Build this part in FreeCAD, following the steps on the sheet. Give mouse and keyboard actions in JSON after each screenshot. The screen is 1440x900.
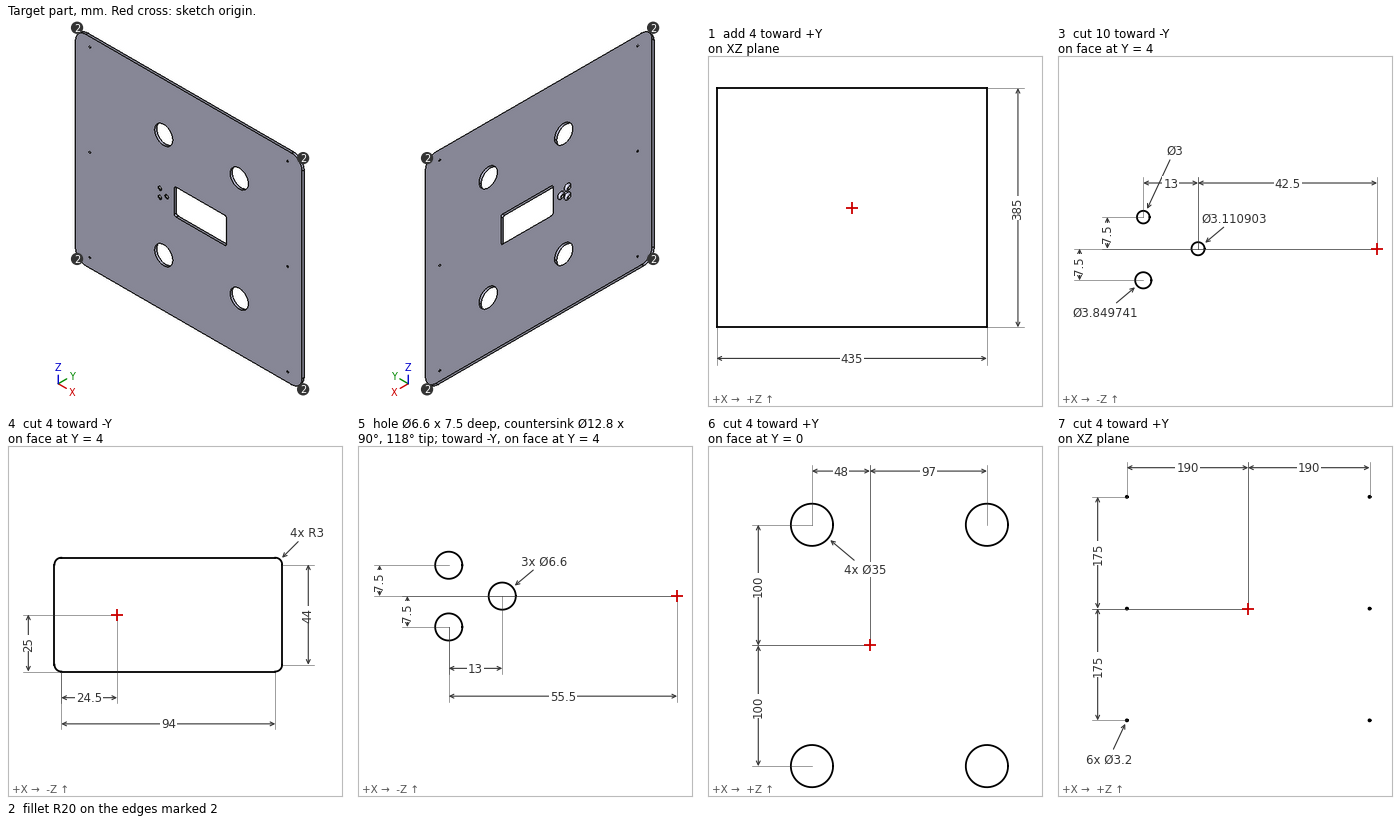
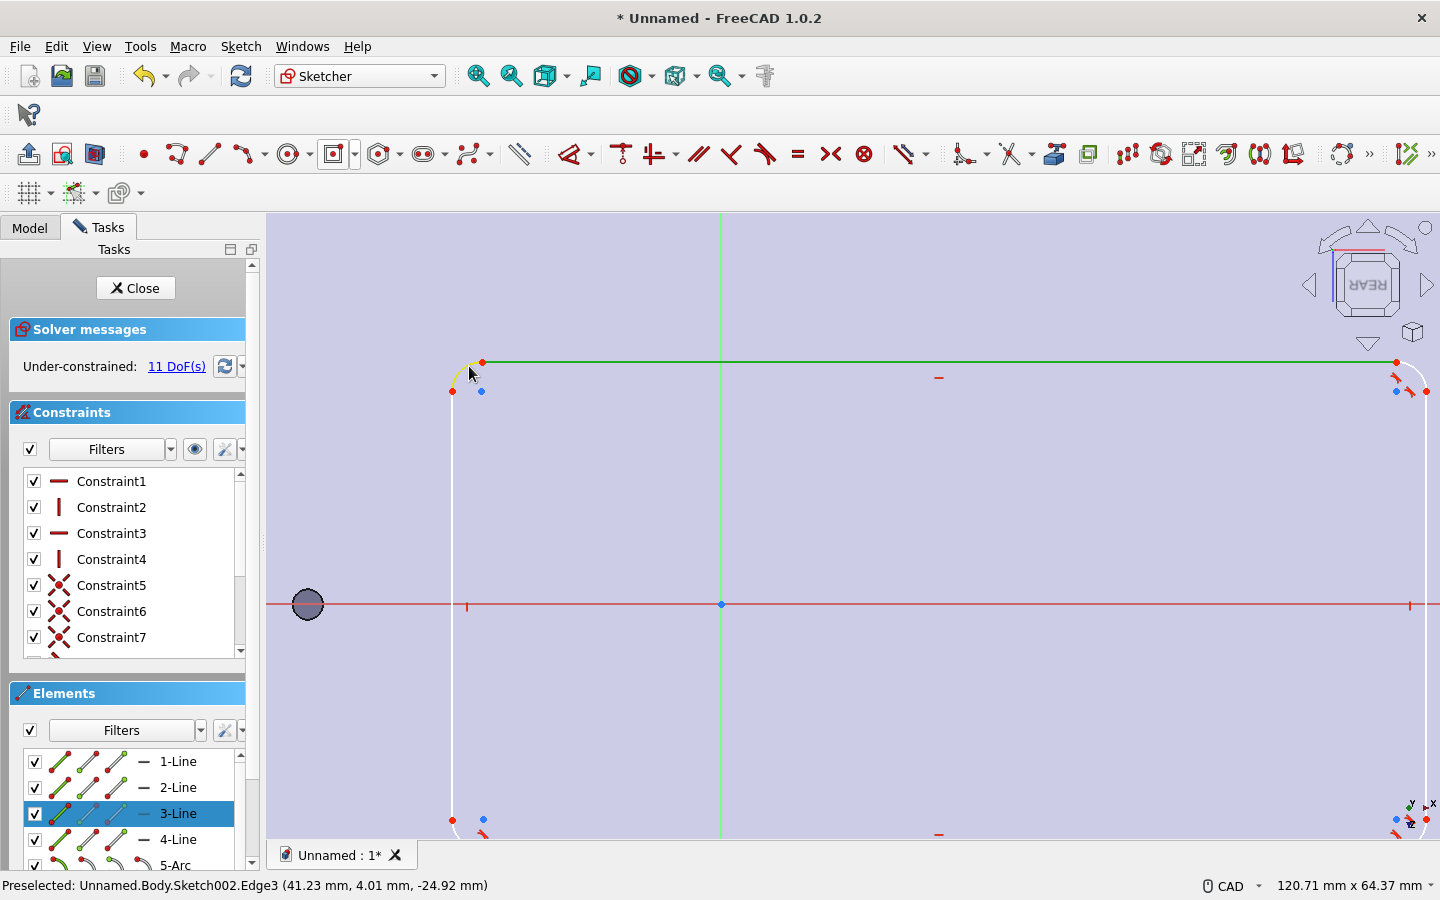
{"action": "left_click", "coordinate": [469, 365]}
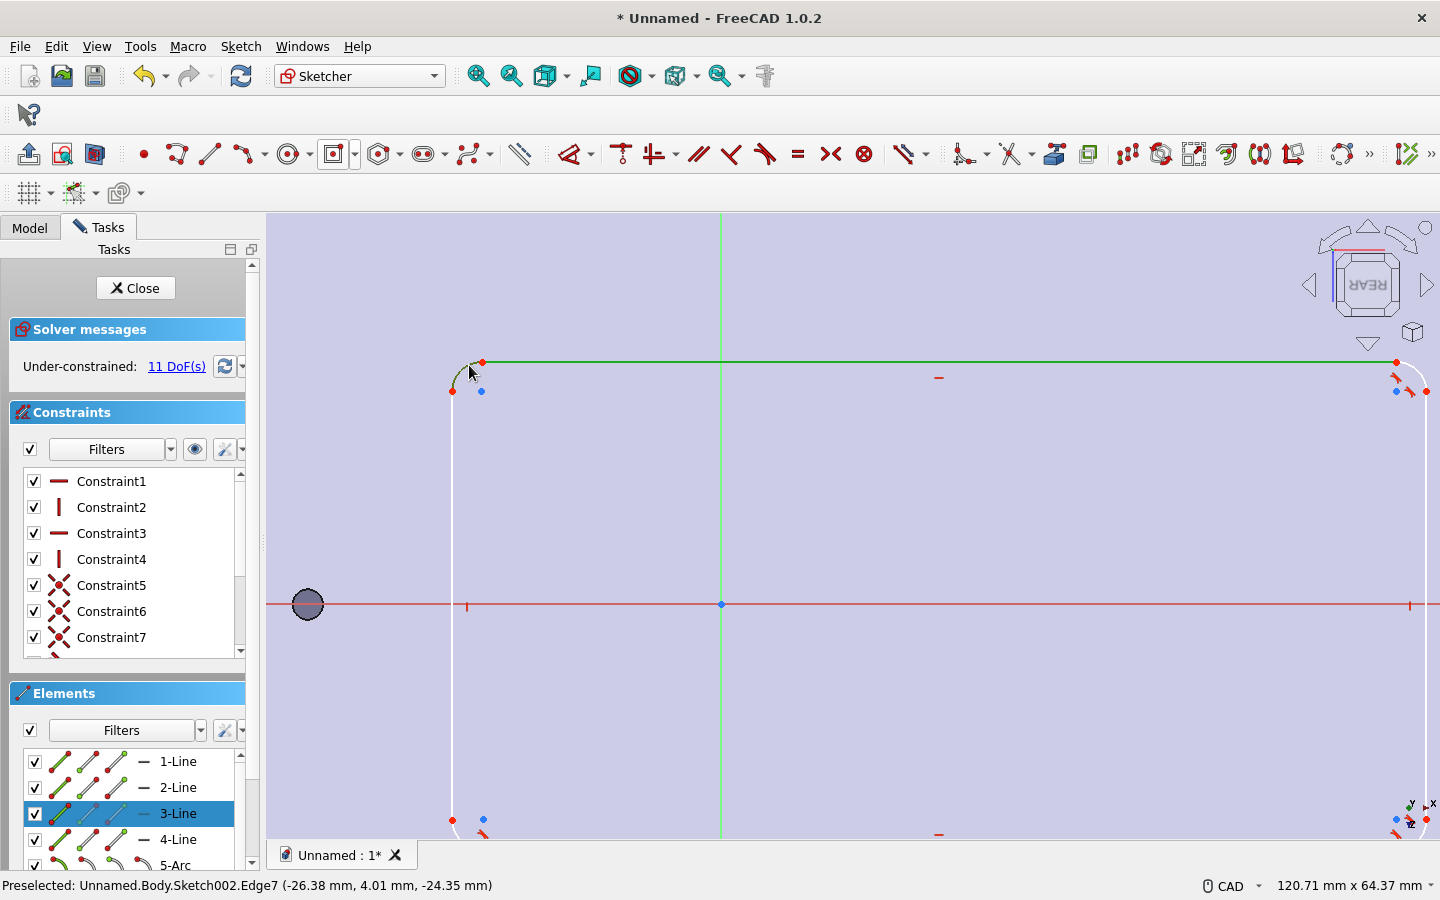
{"action": "left_click", "coordinate": [765, 154]}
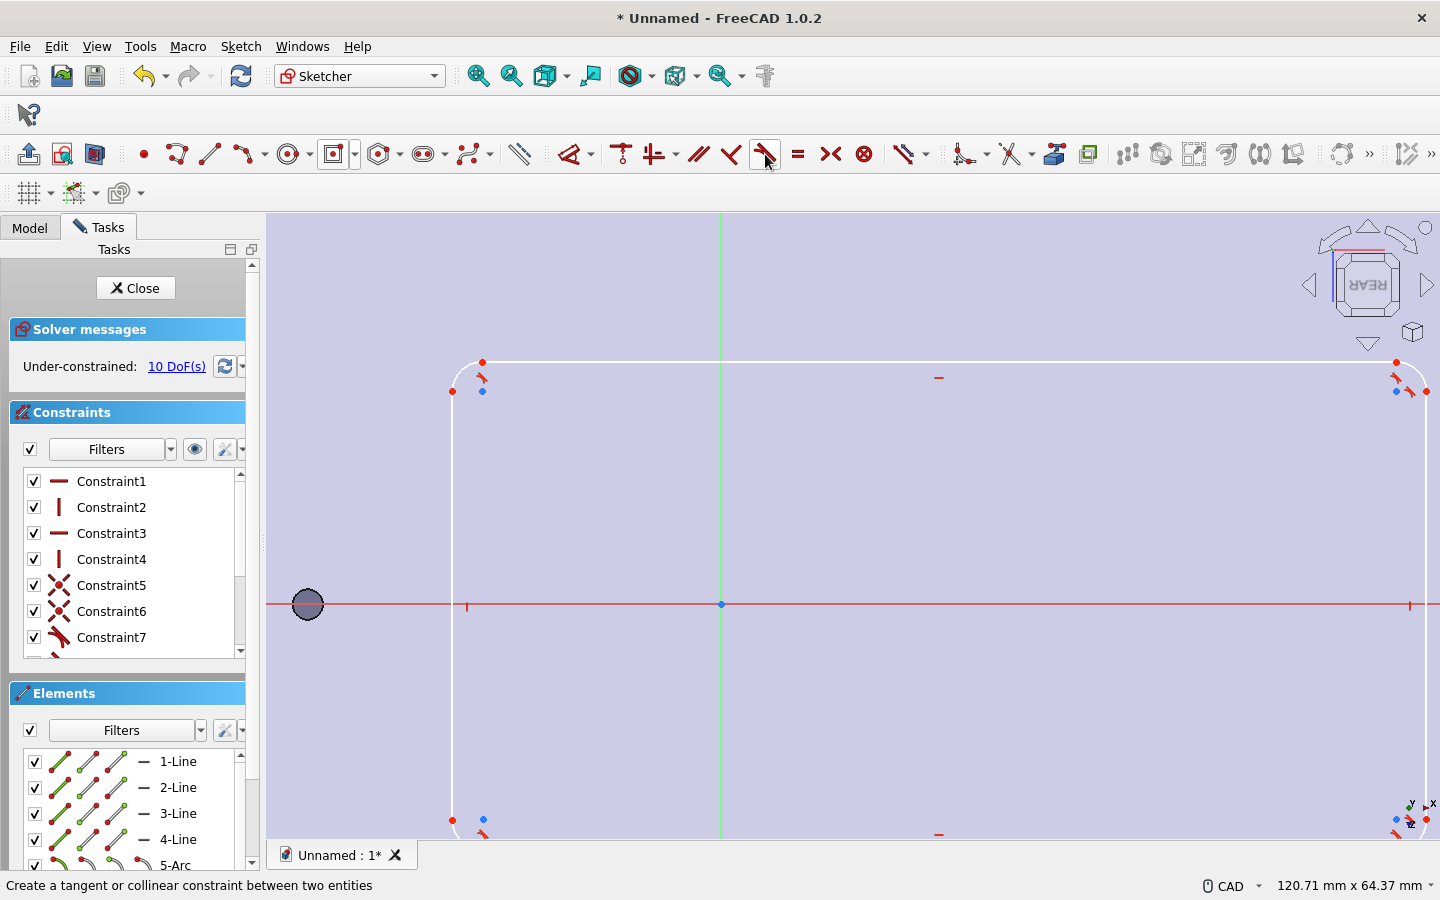
{"action": "left_click", "coordinate": [452, 520]}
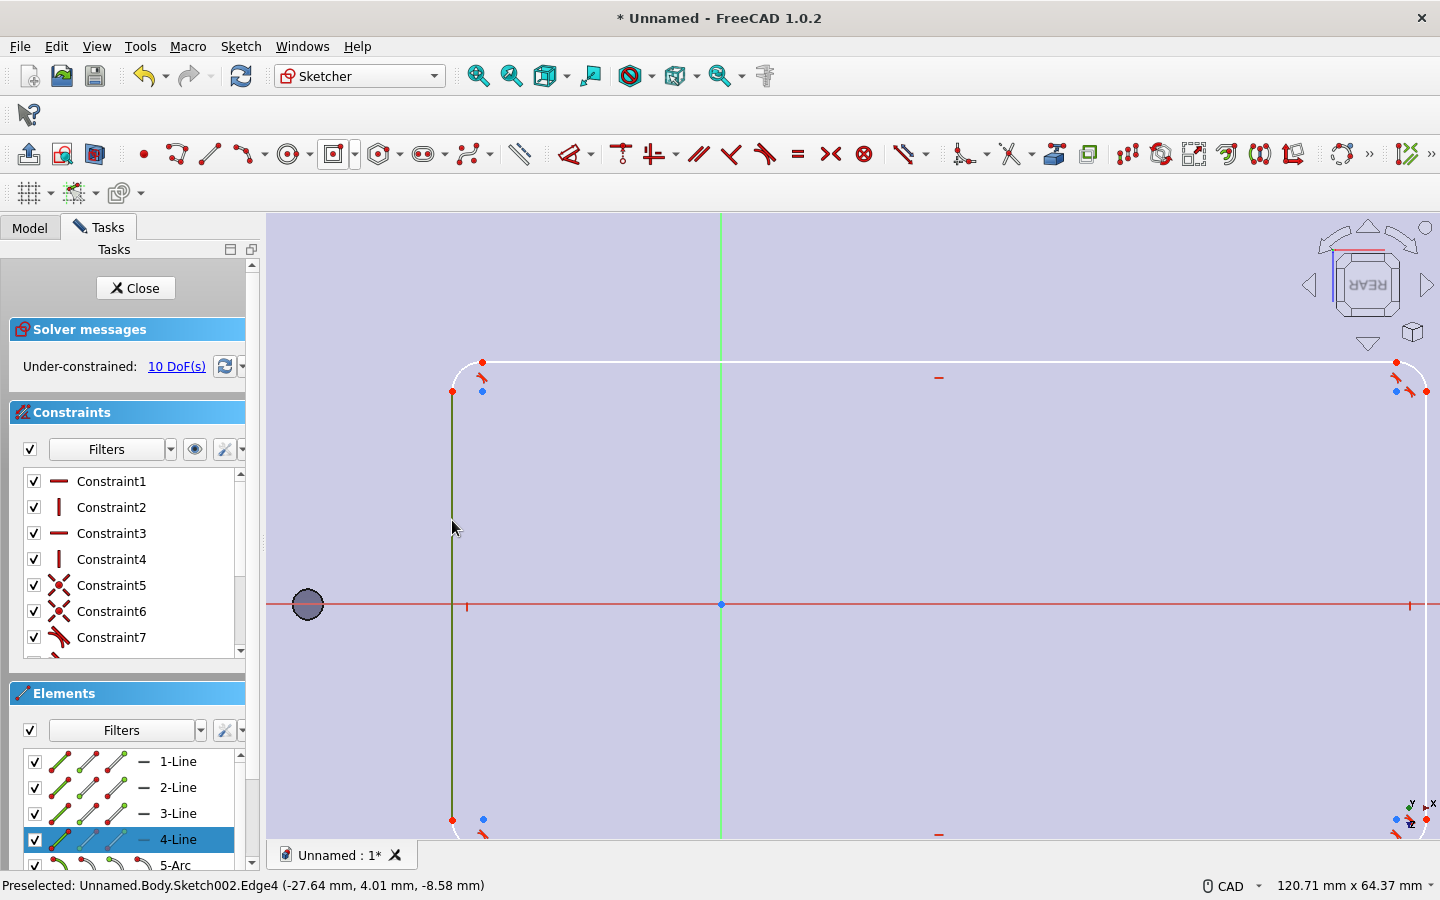
{"action": "left_click", "coordinate": [469, 365]}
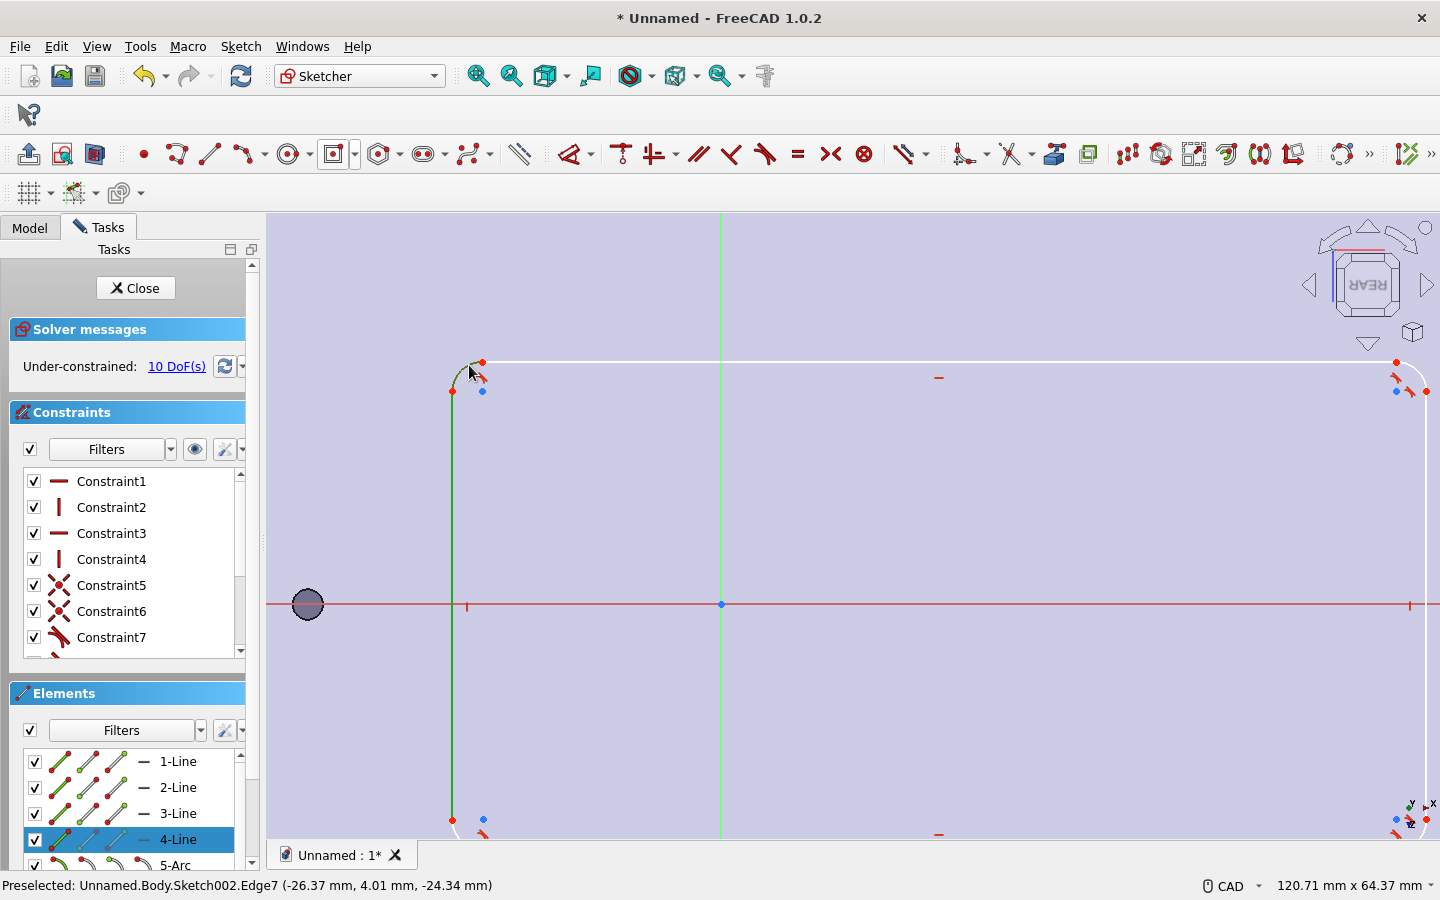
{"action": "left_click", "coordinate": [765, 154]}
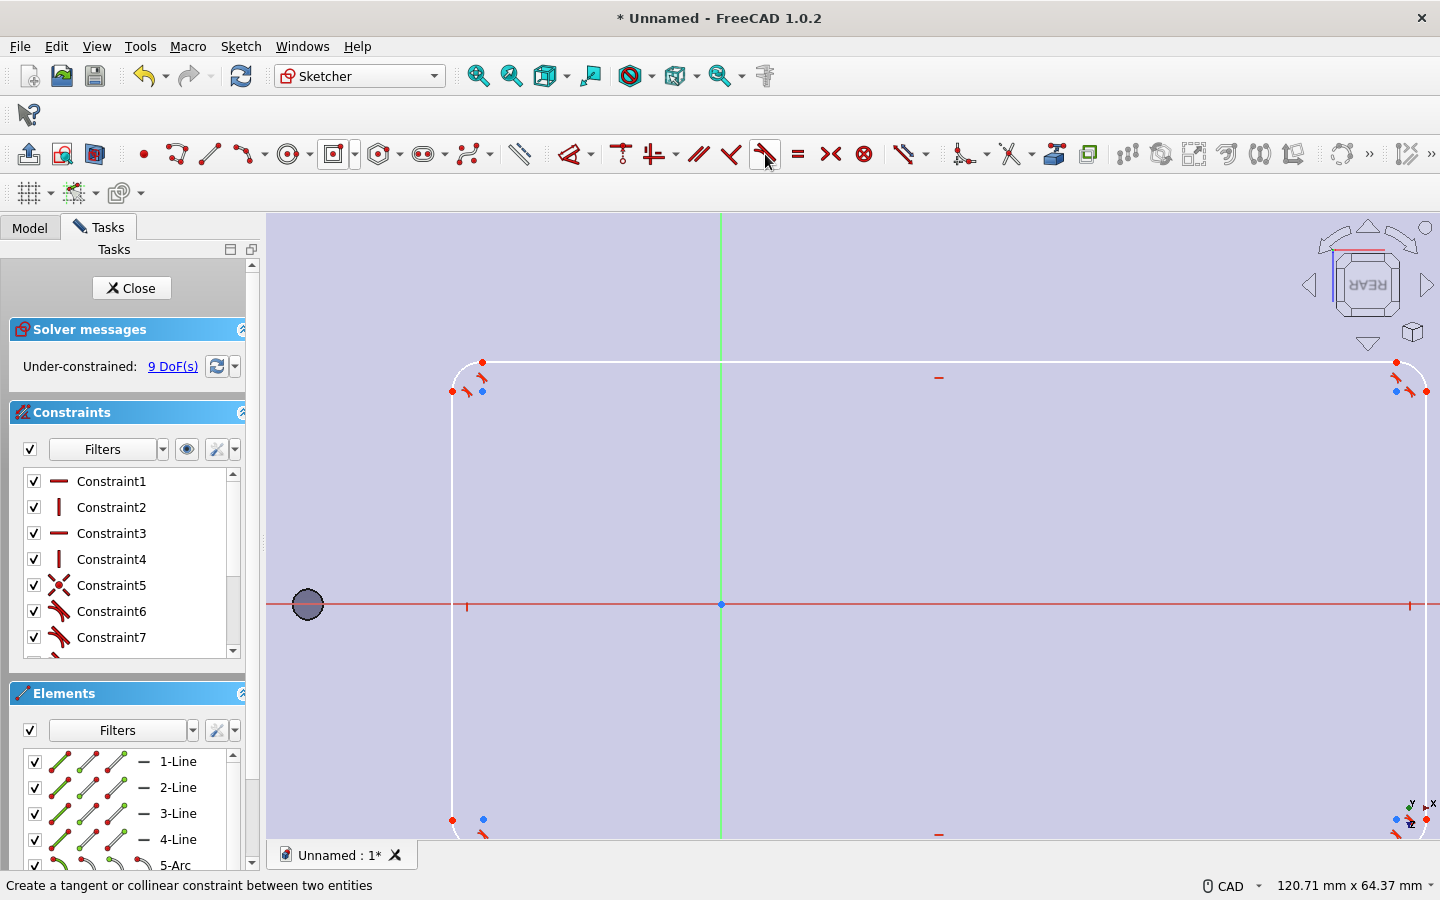
{"action": "left_click", "coordinate": [452, 520]}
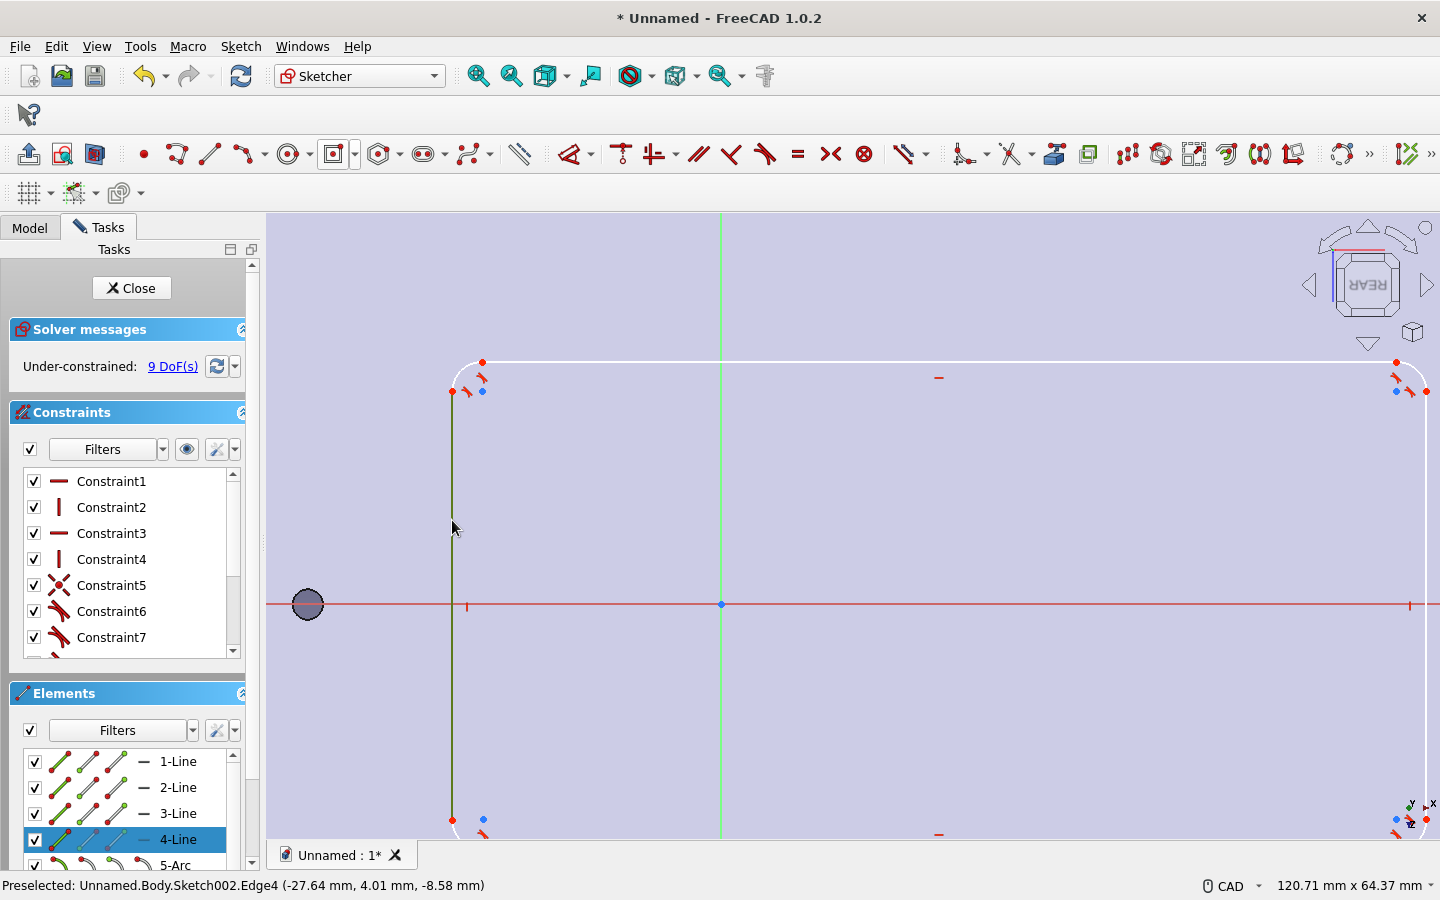
{"action": "scroll", "coordinate": [468, 366], "scroll_direction": "down", "scroll_amount": 2}